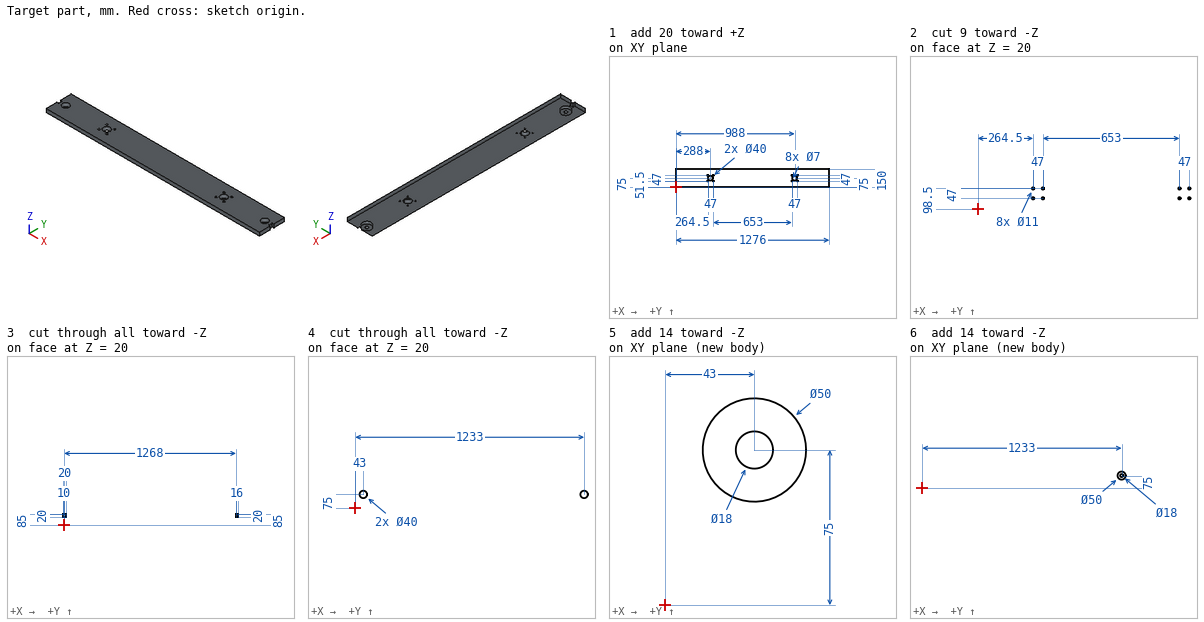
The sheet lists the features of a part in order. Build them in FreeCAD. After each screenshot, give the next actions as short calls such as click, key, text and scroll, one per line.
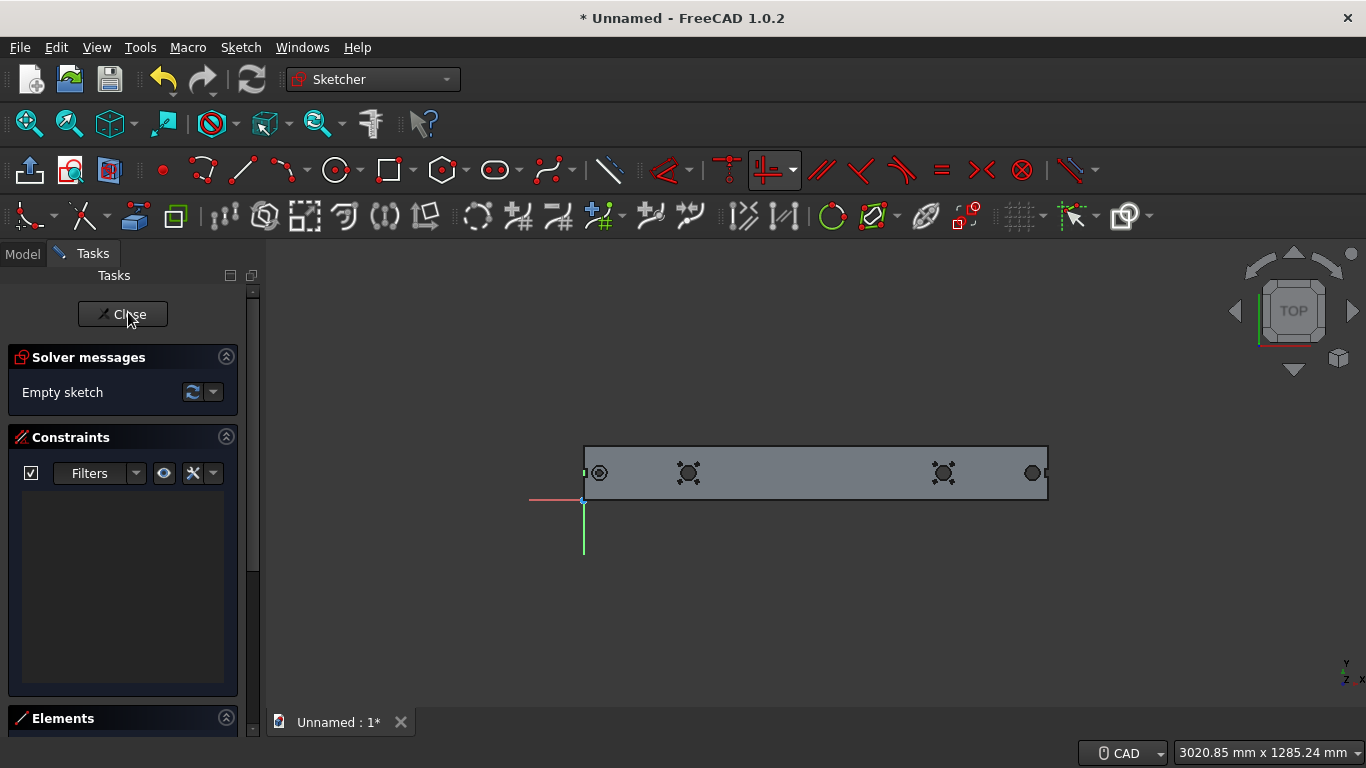
scroll(1051, 473, up, 14)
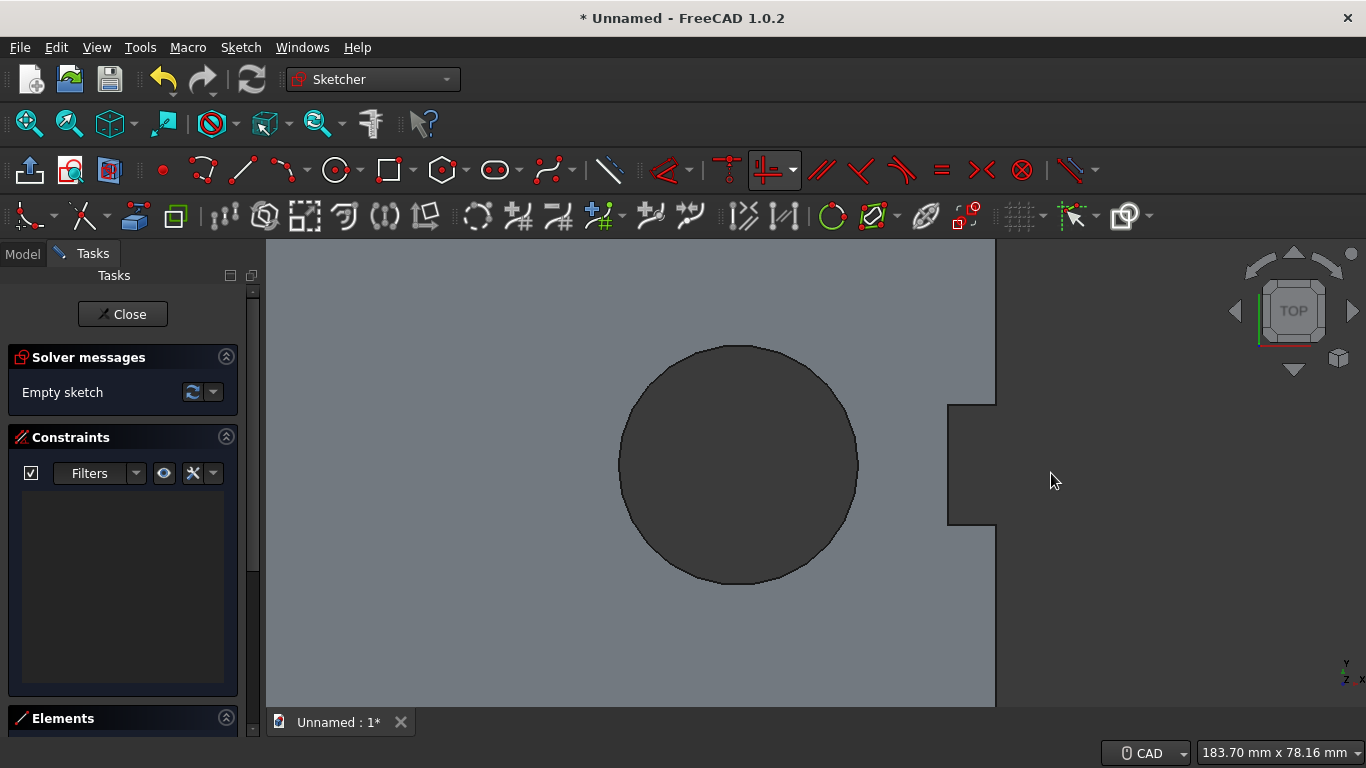
click(336, 170)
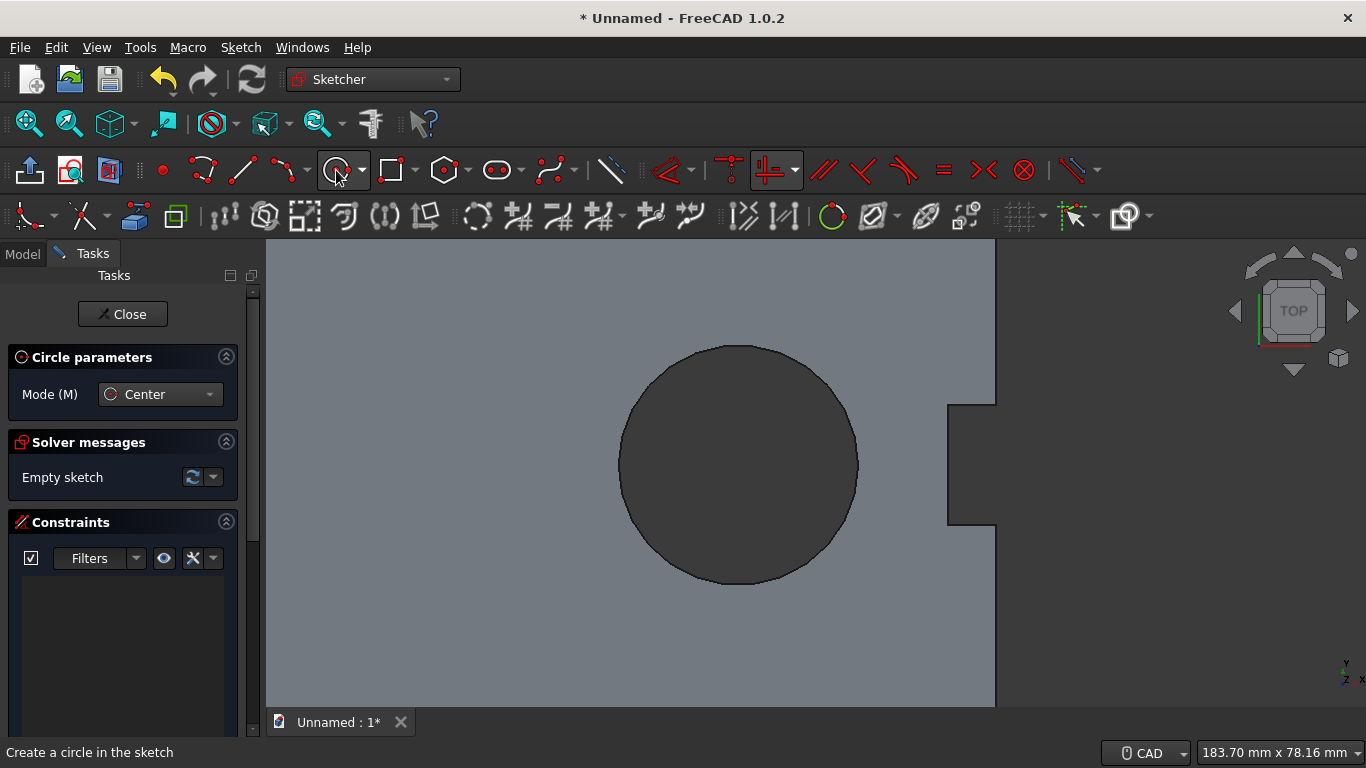
click(738, 465)
move(844, 359)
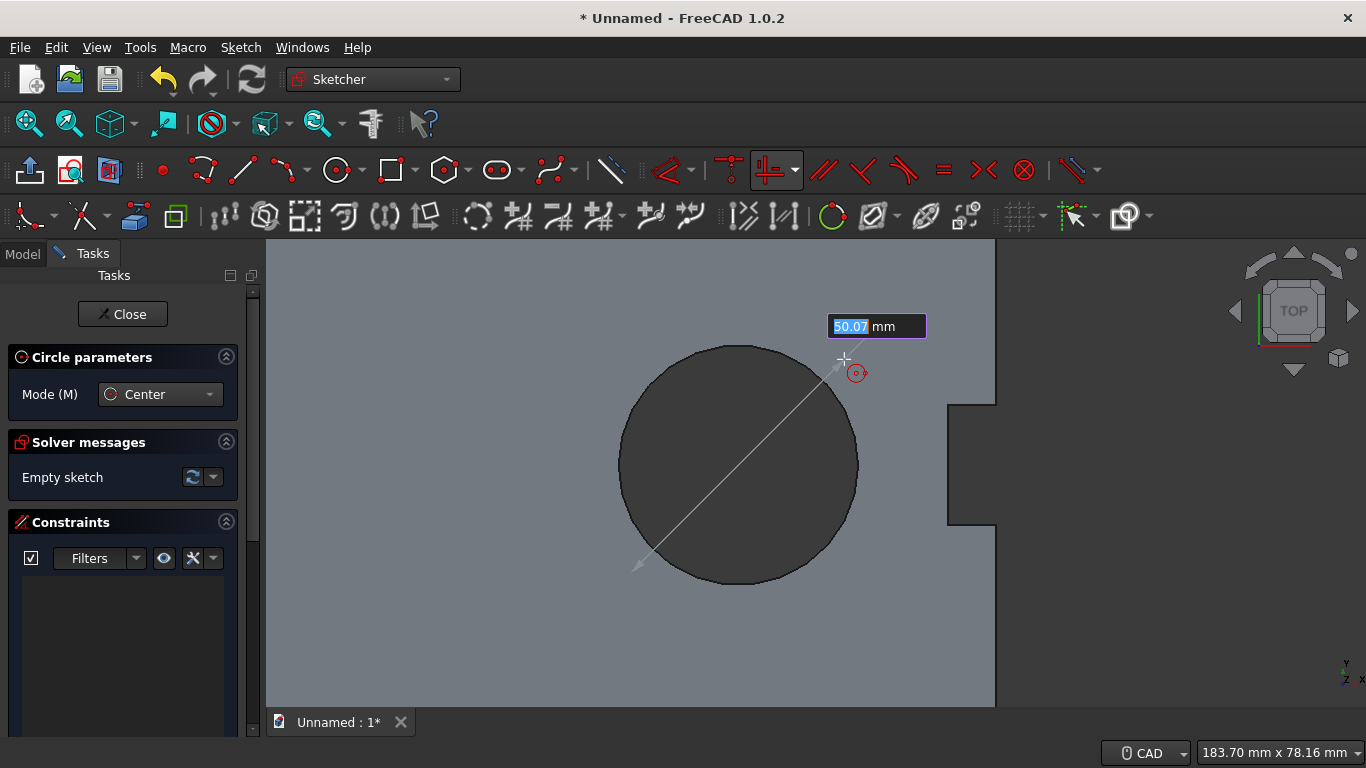
text(50)
key(Return)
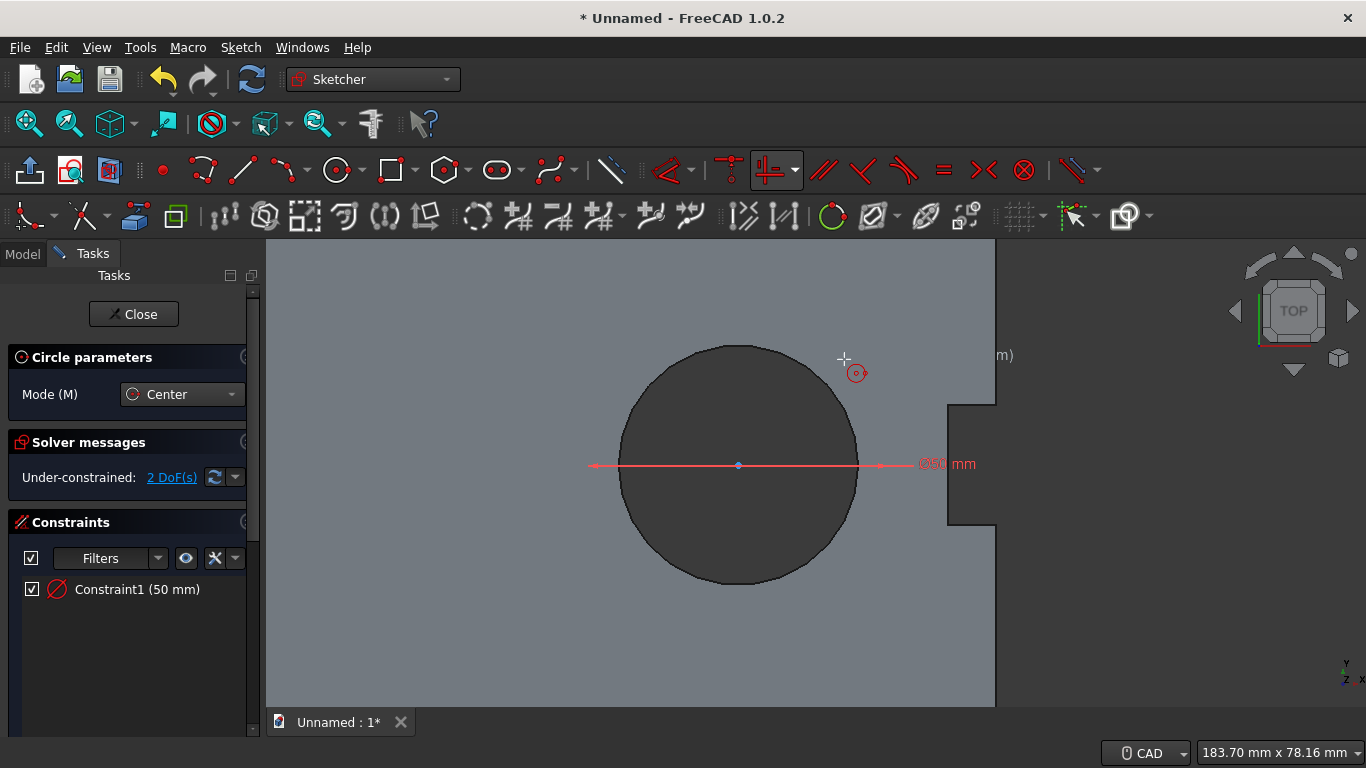
click(738, 466)
move(776, 427)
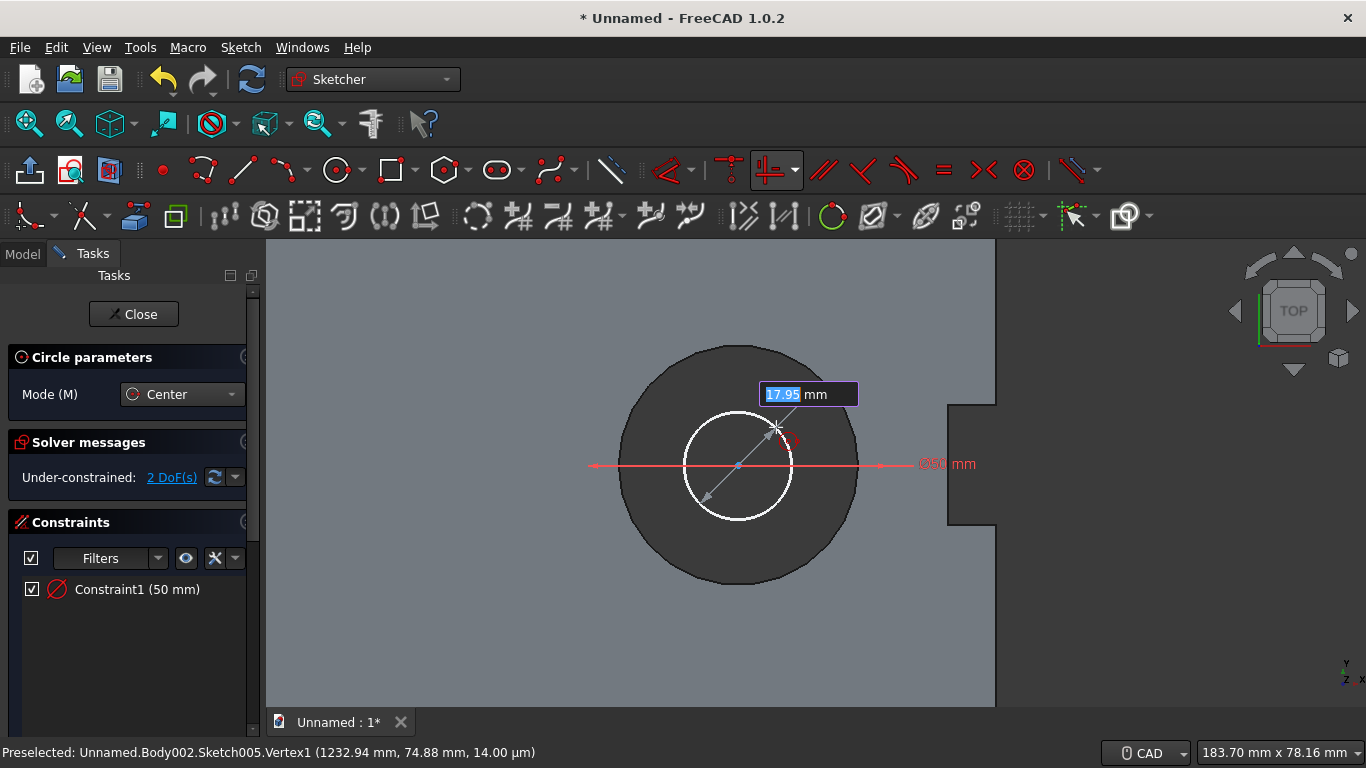
text(18)
key(Return)
key(Escape)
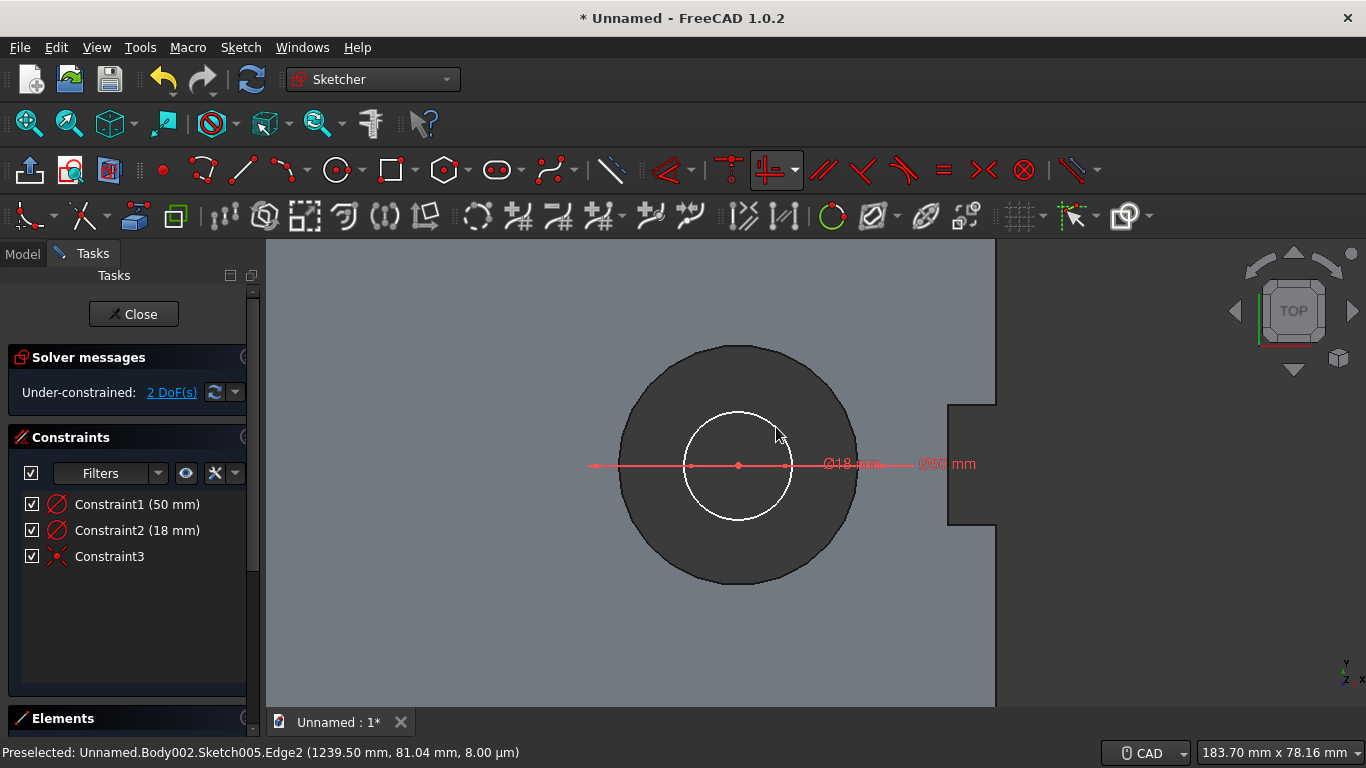
click(666, 170)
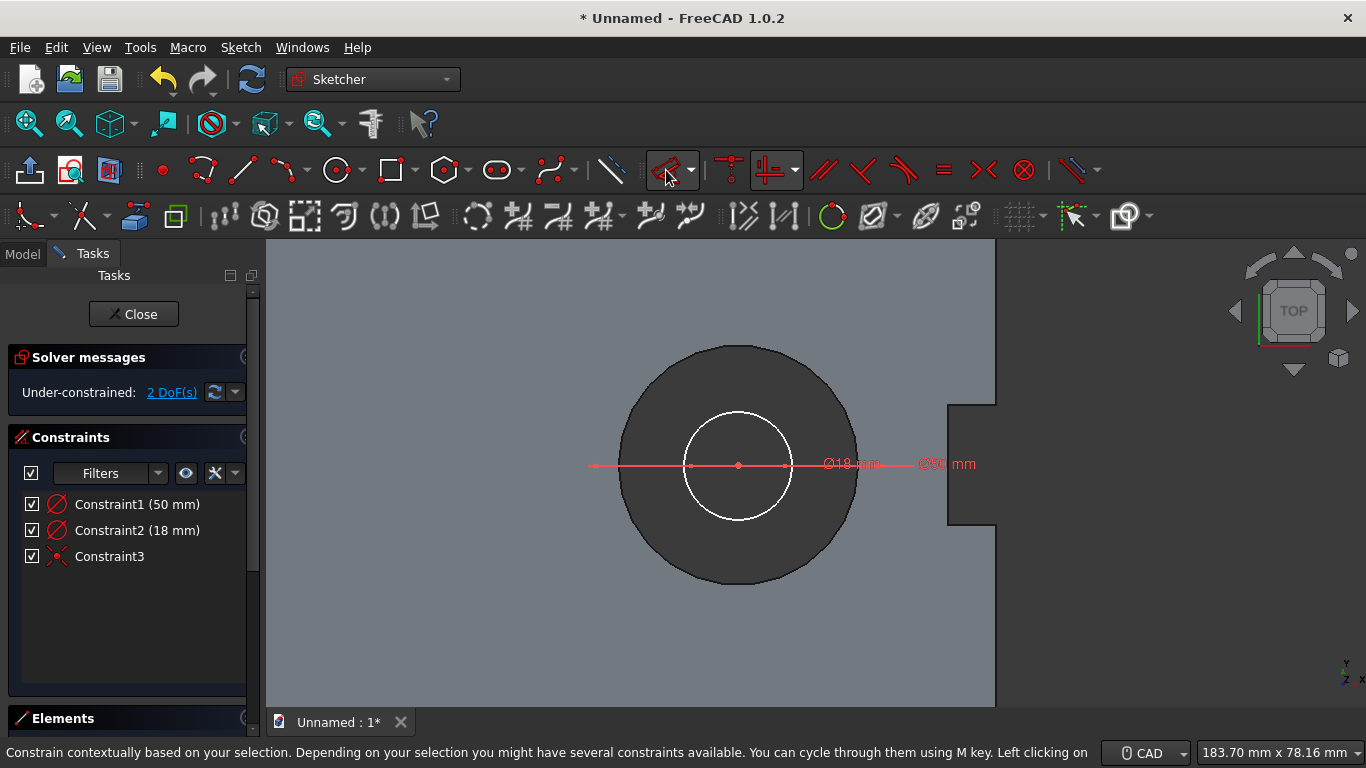
click(738, 466)
click(772, 572)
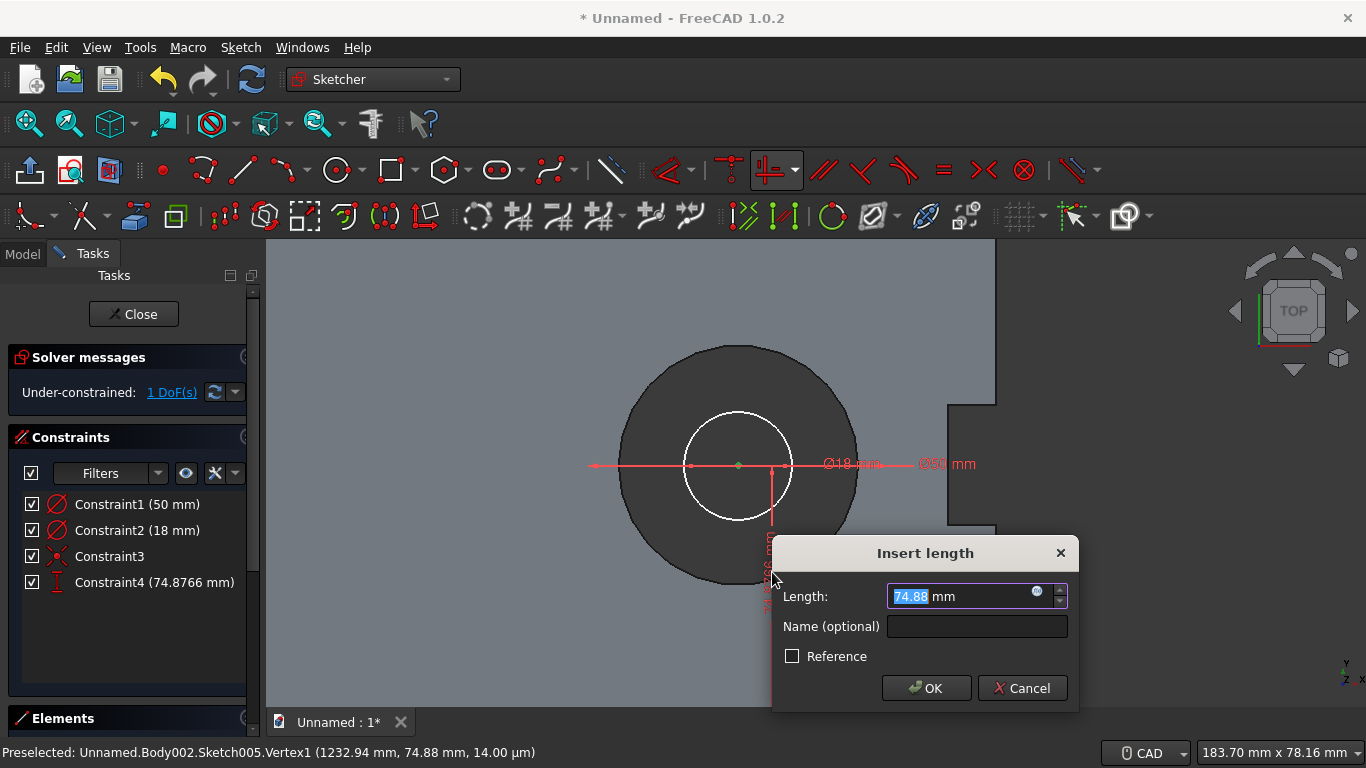
text(75)
key(Return)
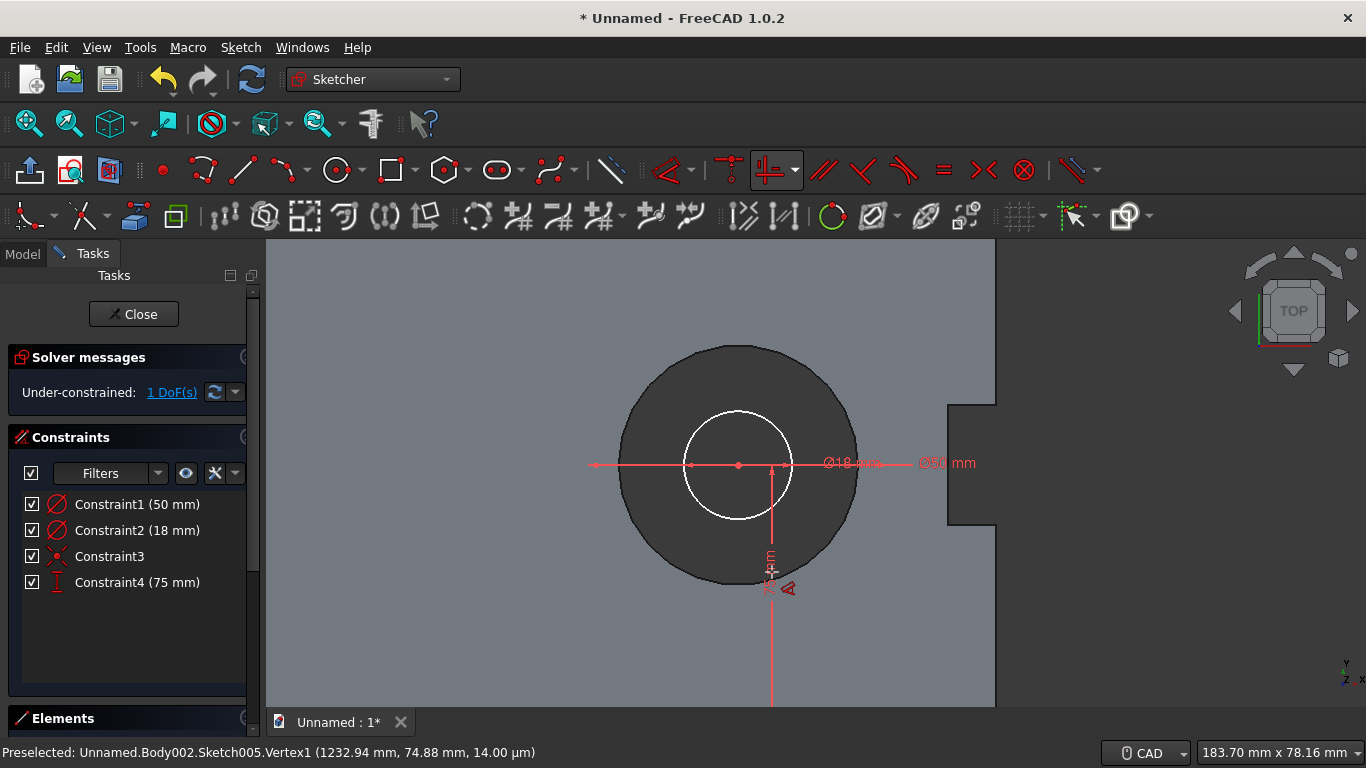
click(738, 465)
click(516, 431)